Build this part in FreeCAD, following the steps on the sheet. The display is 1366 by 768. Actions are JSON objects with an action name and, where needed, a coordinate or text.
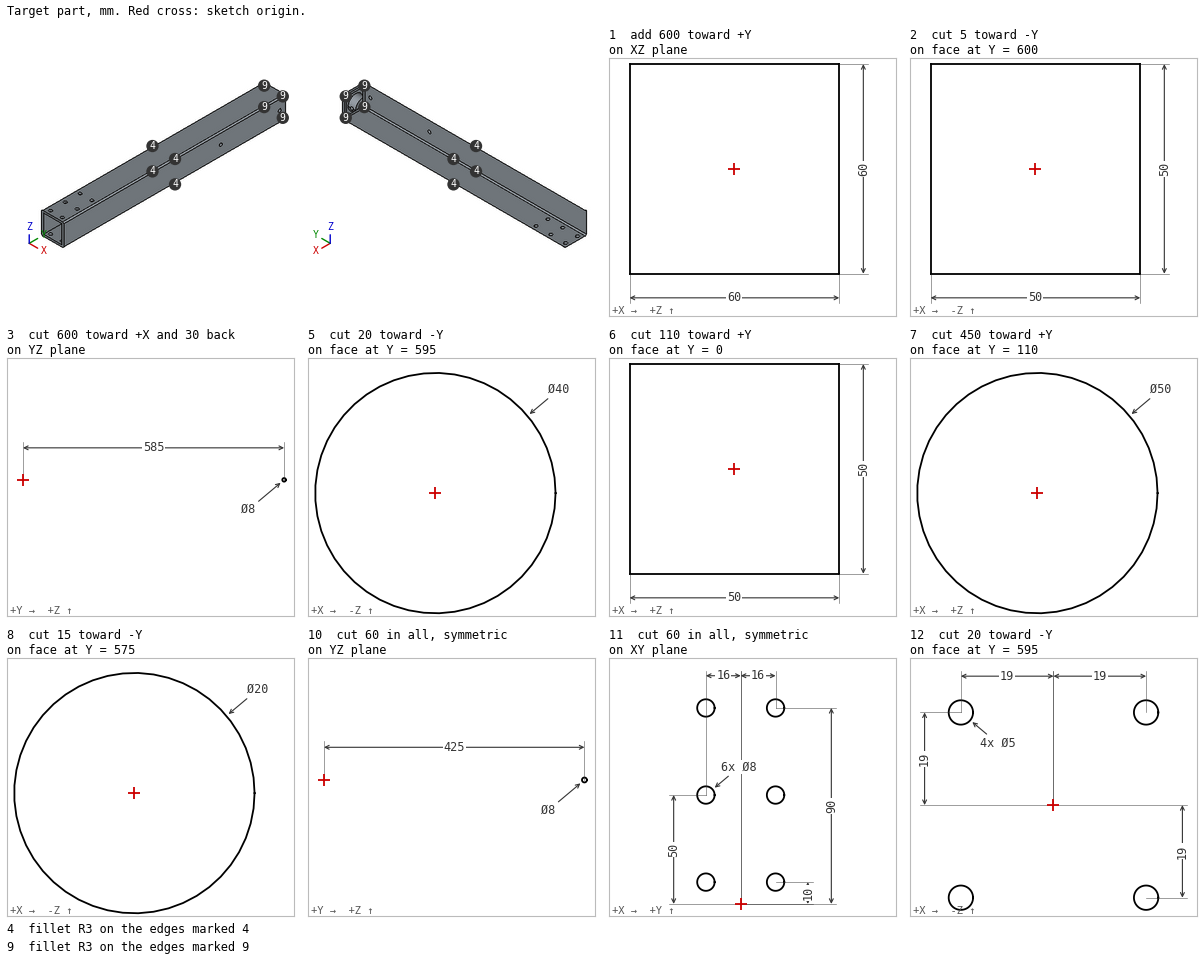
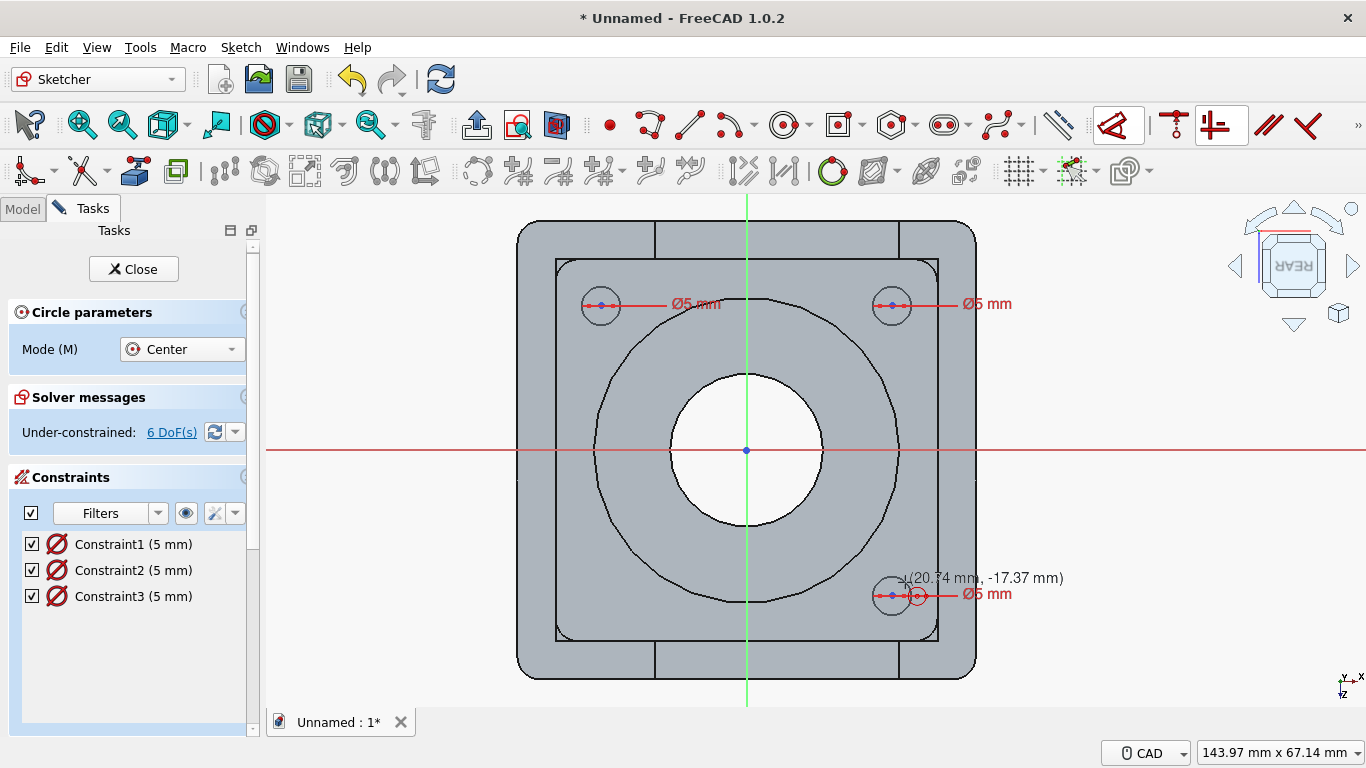
{"action": "left_click", "coordinate": [601, 595]}
{"action": "mouse_move", "coordinate": [615, 582]}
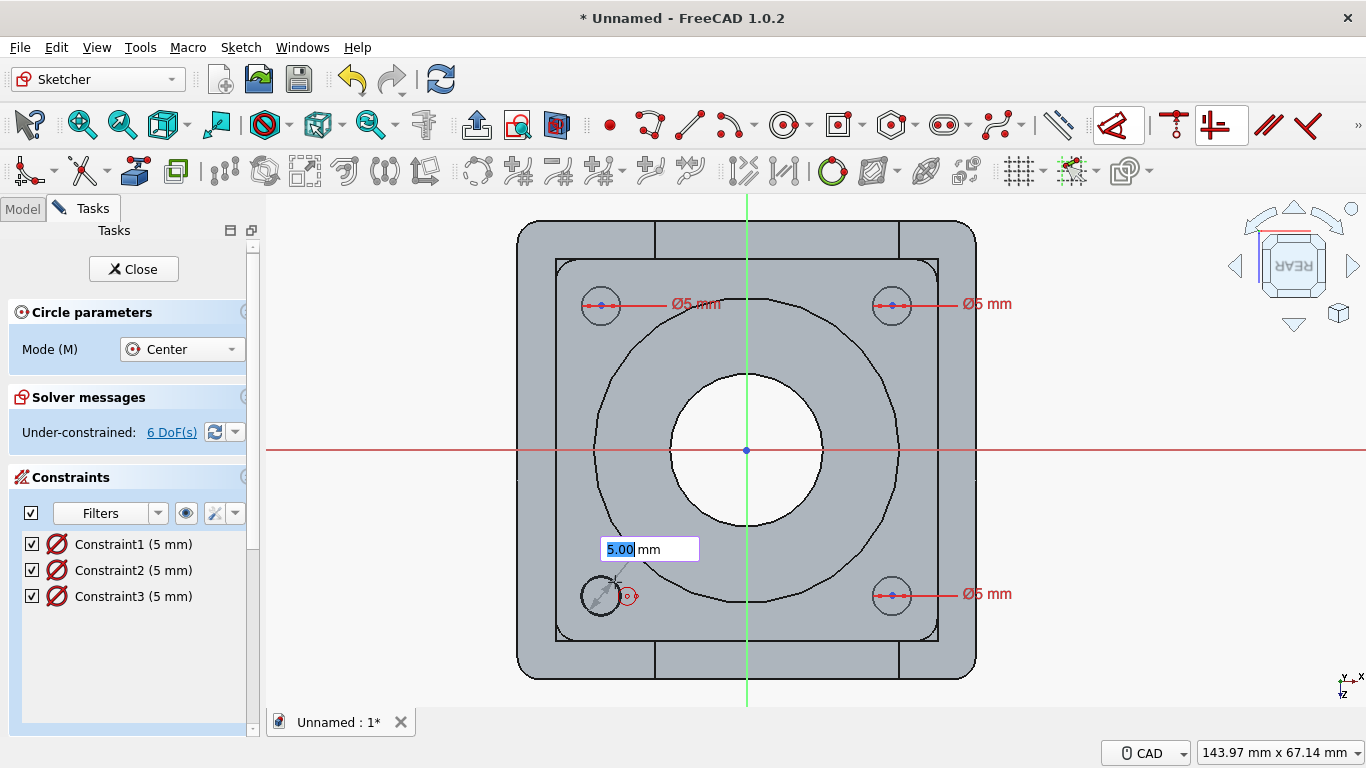
{"action": "type", "text": "5"}
{"action": "key", "text": "Return"}
{"action": "key", "text": "Escape"}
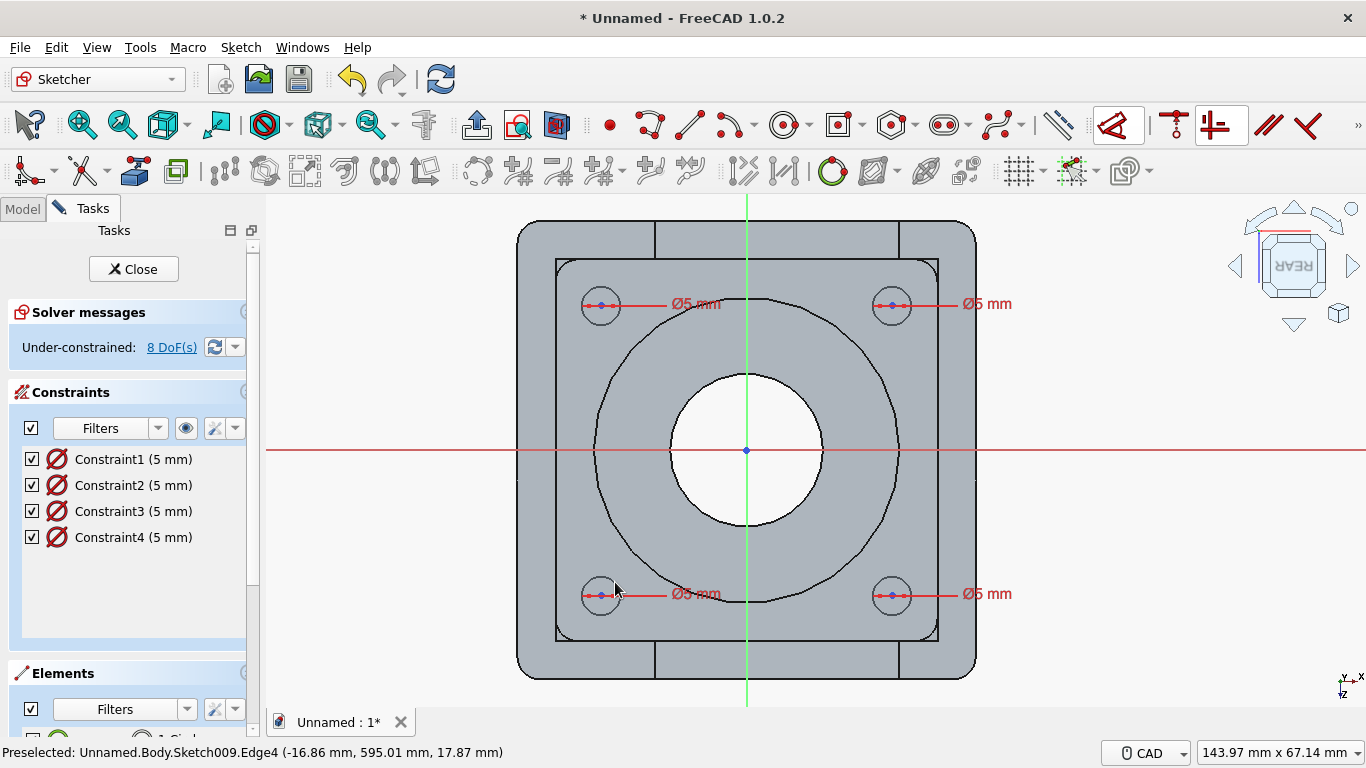
{"action": "left_click", "coordinate": [601, 306]}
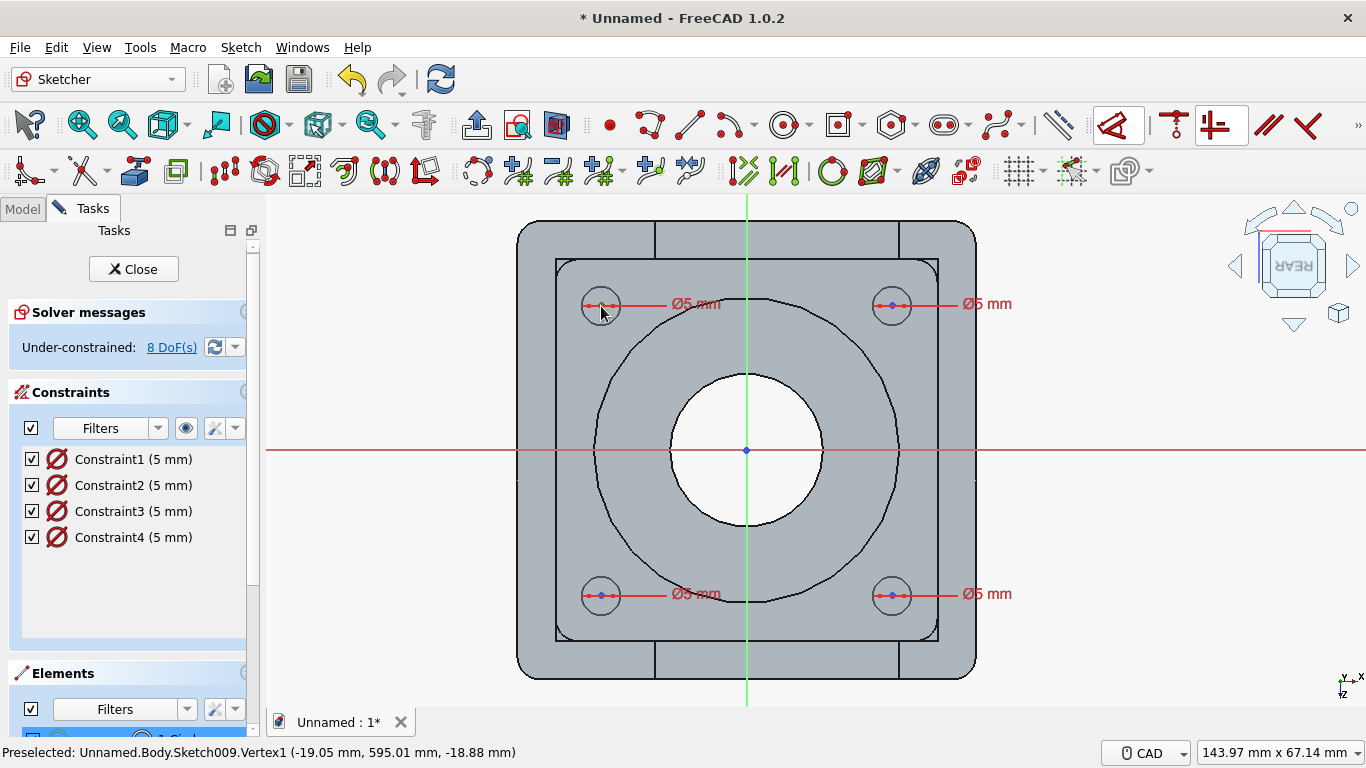
{"action": "left_click", "coordinate": [892, 306]}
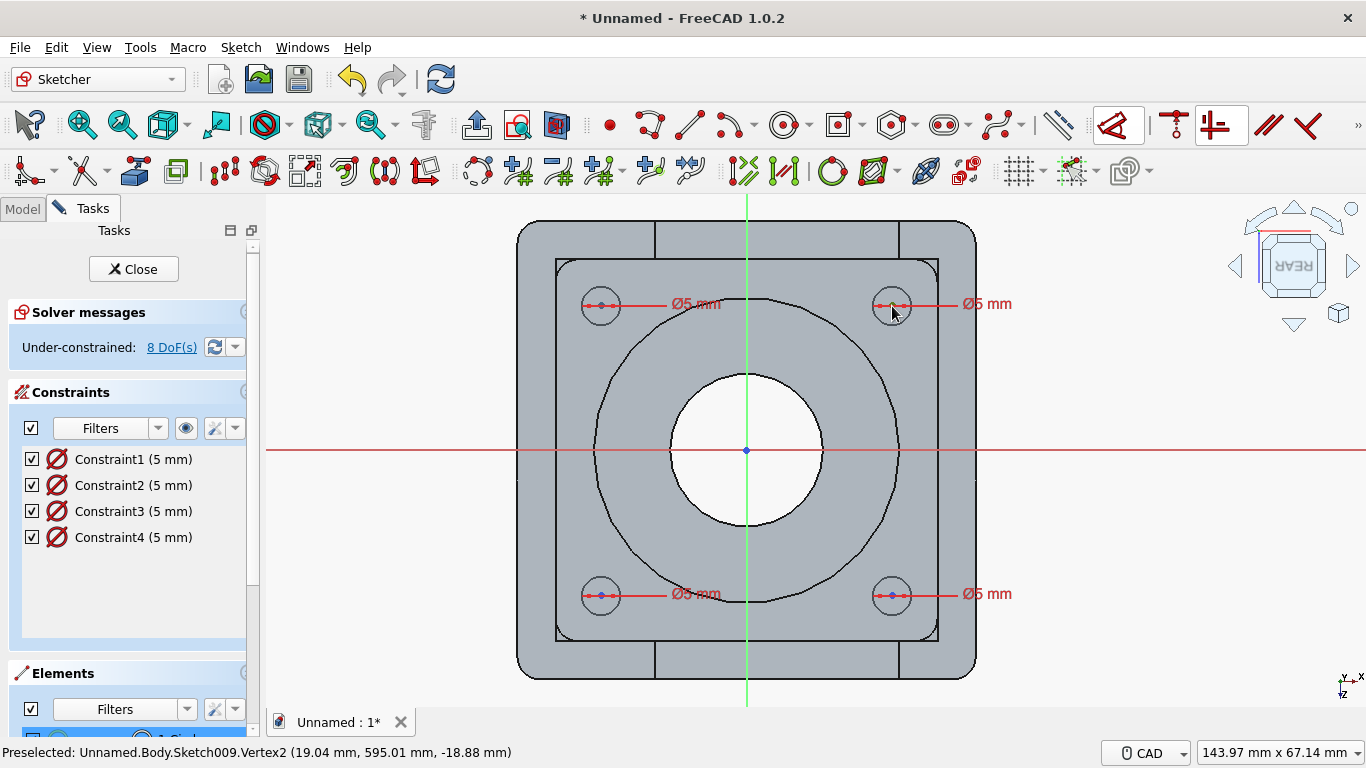
{"action": "left_click", "coordinate": [1242, 126]}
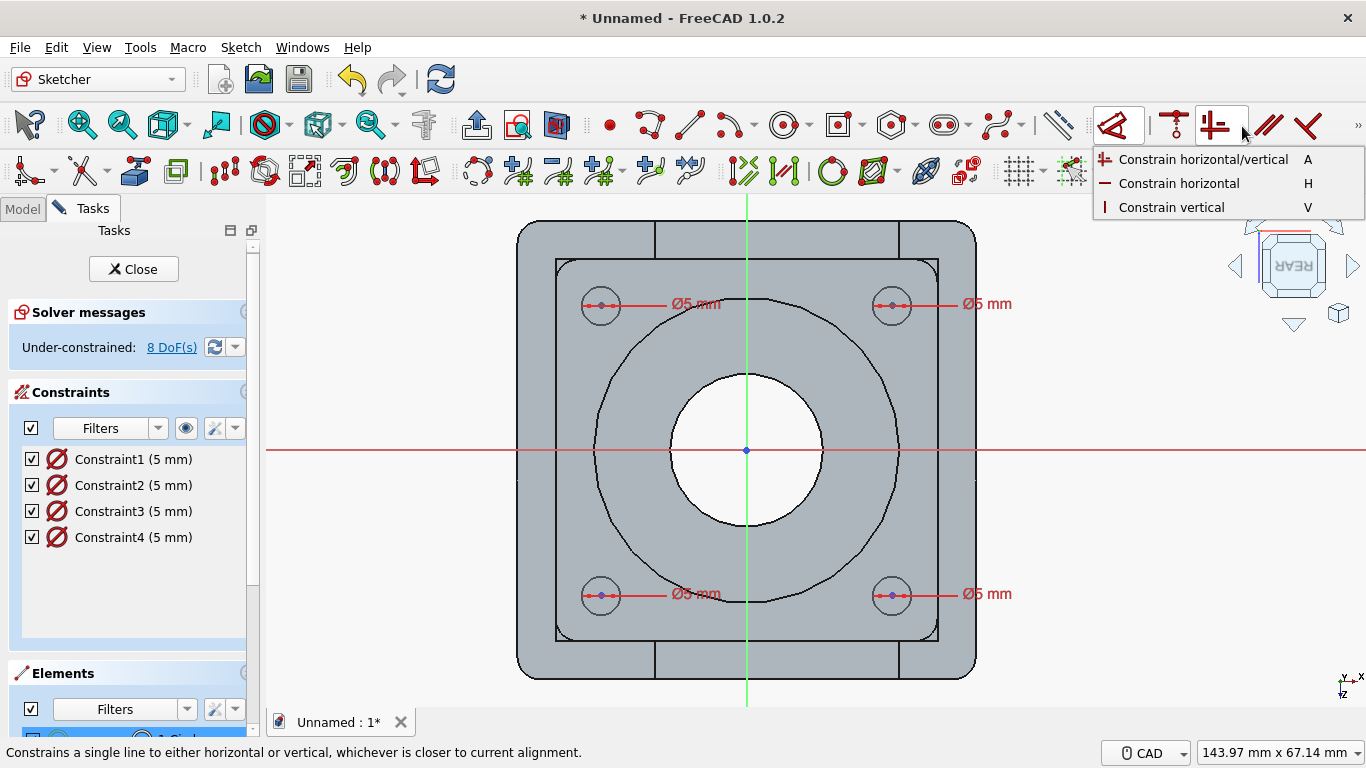
{"action": "left_click", "coordinate": [1229, 183]}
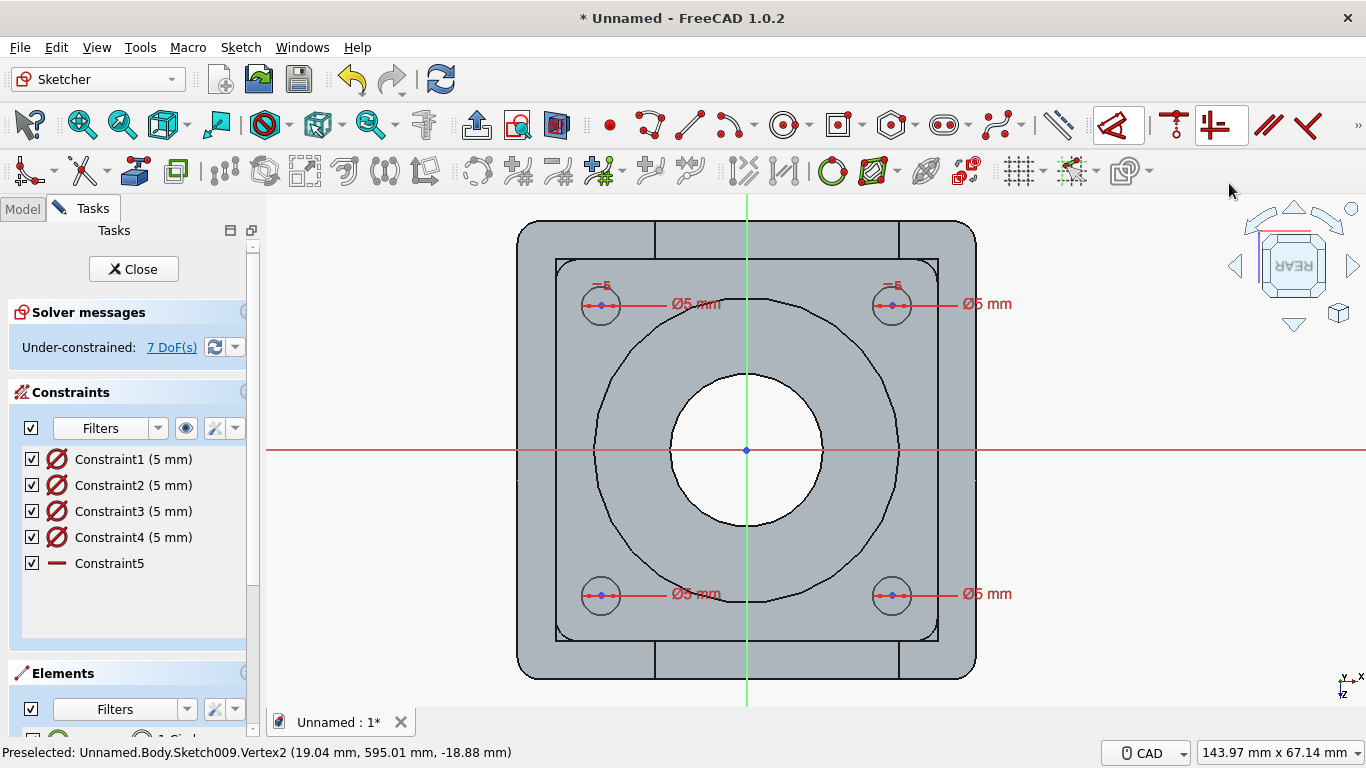
{"action": "left_click", "coordinate": [892, 306]}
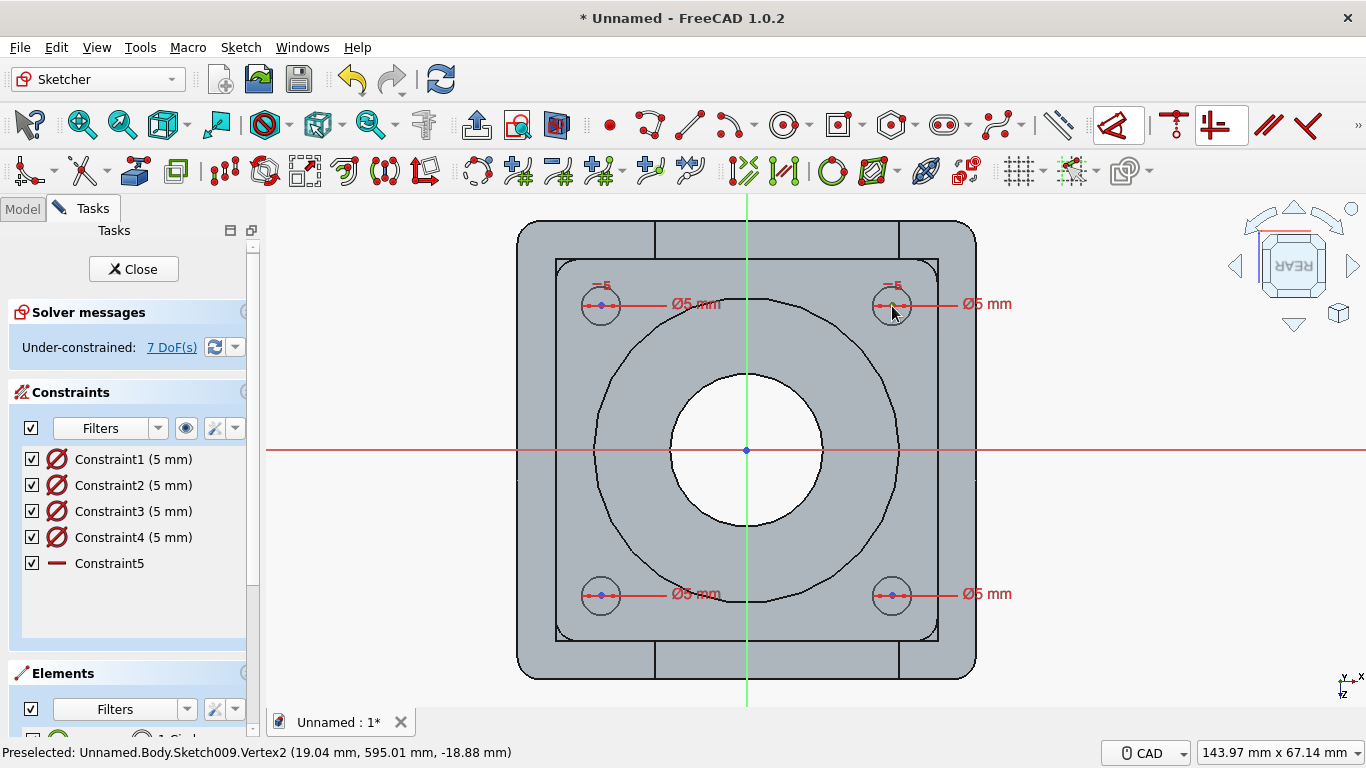
{"action": "left_click", "coordinate": [892, 596]}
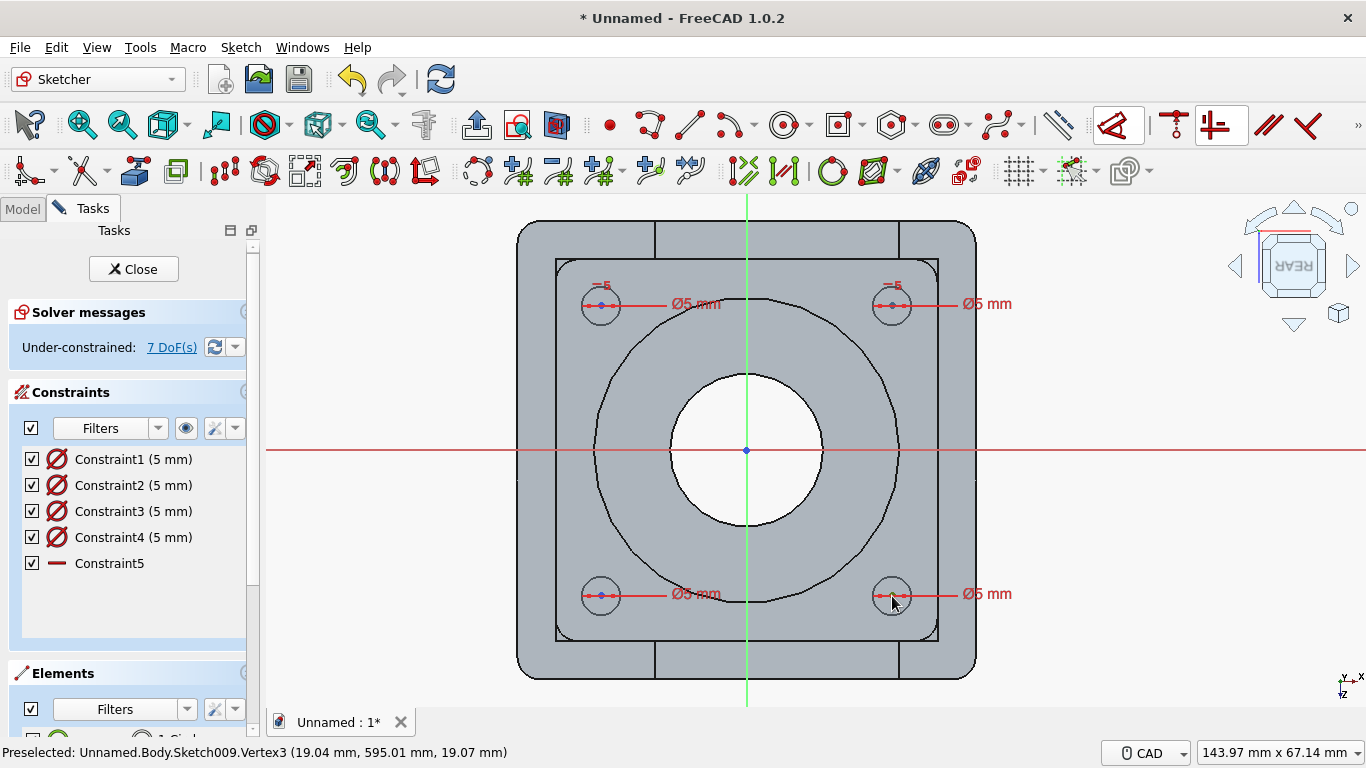
{"action": "left_click", "coordinate": [1242, 126]}